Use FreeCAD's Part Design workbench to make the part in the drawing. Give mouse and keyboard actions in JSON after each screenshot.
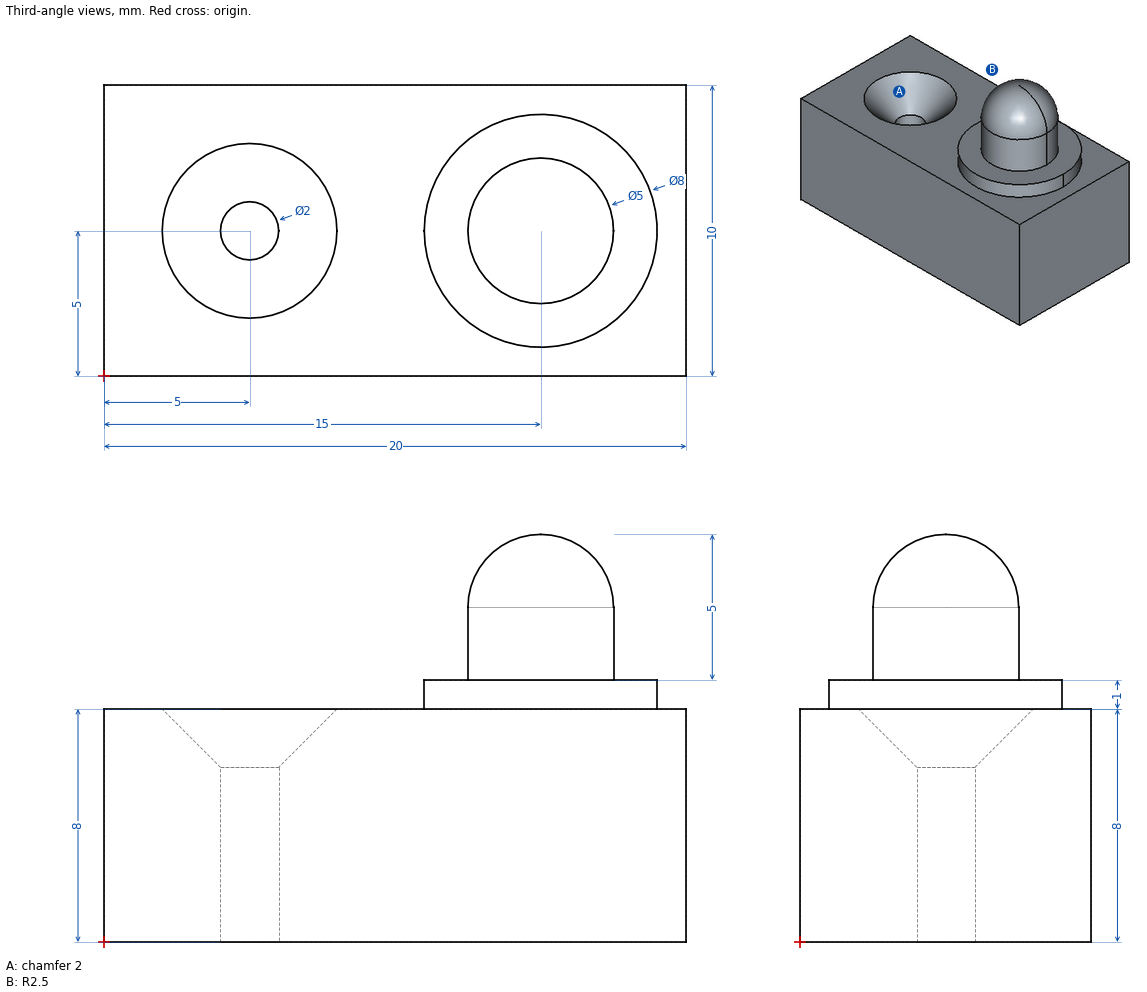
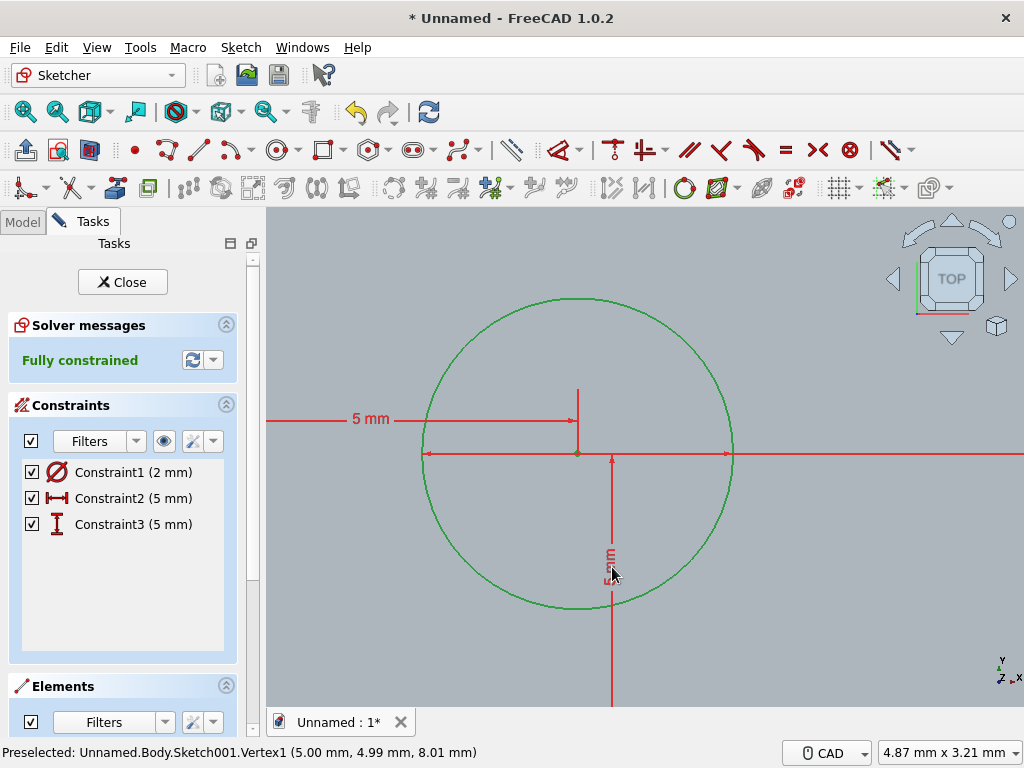
{"action": "left_click", "coordinate": [123, 282]}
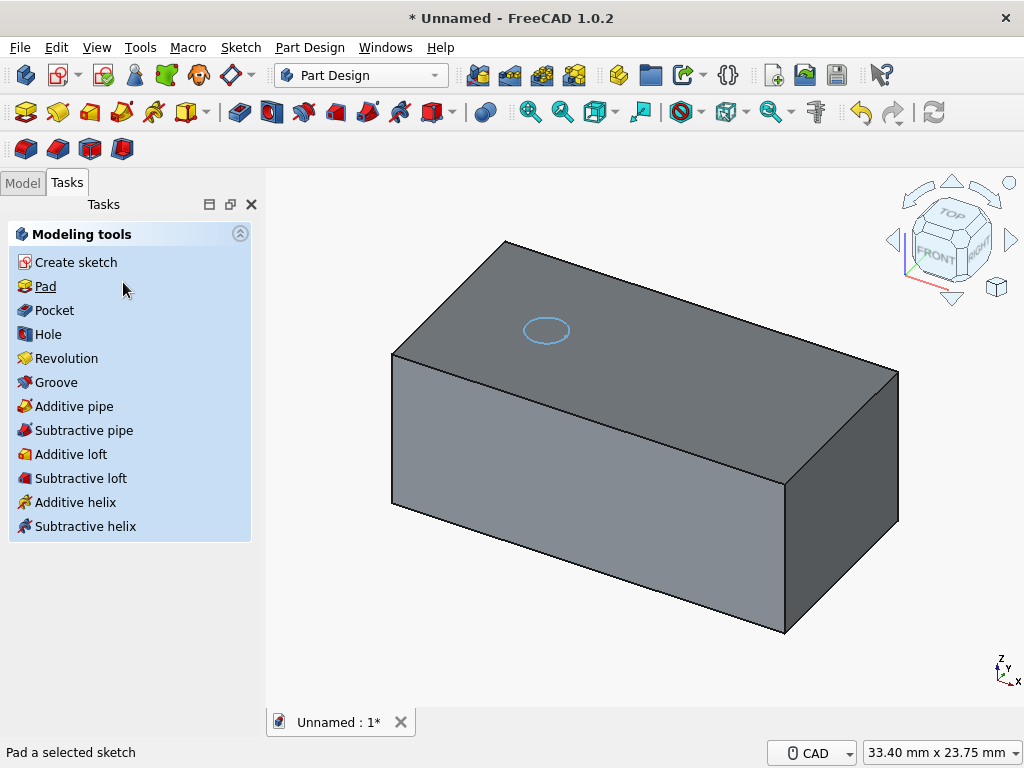
{"action": "left_click", "coordinate": [240, 112]}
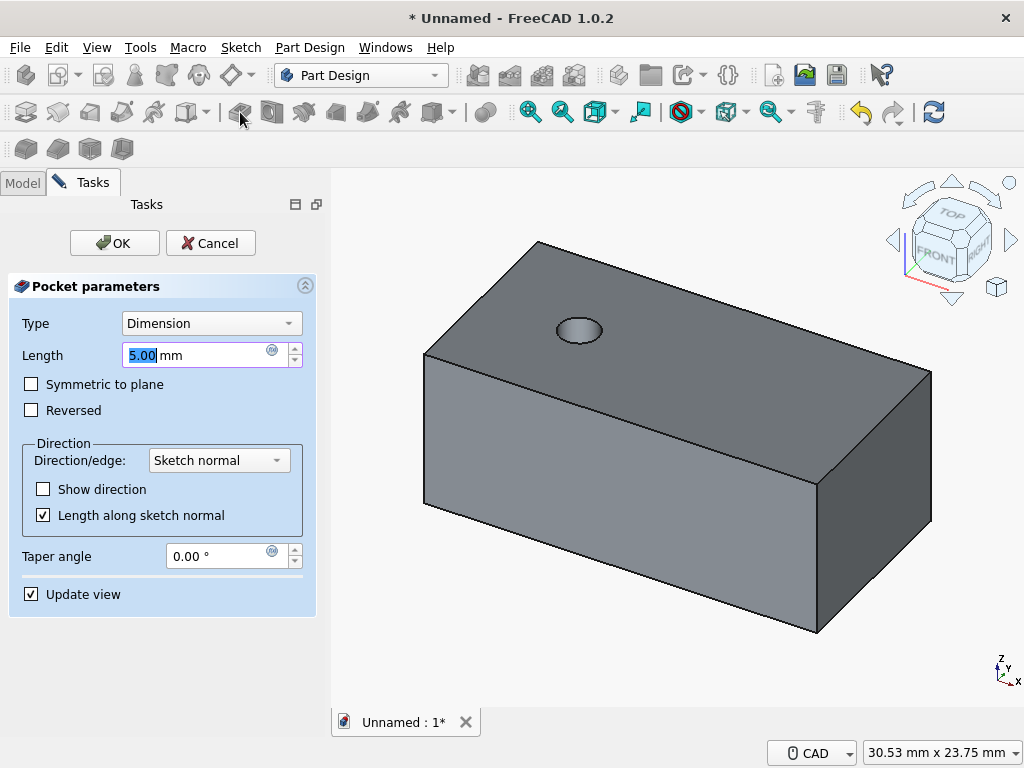
{"action": "type", "text": "8"}
{"action": "key", "text": "Tab"}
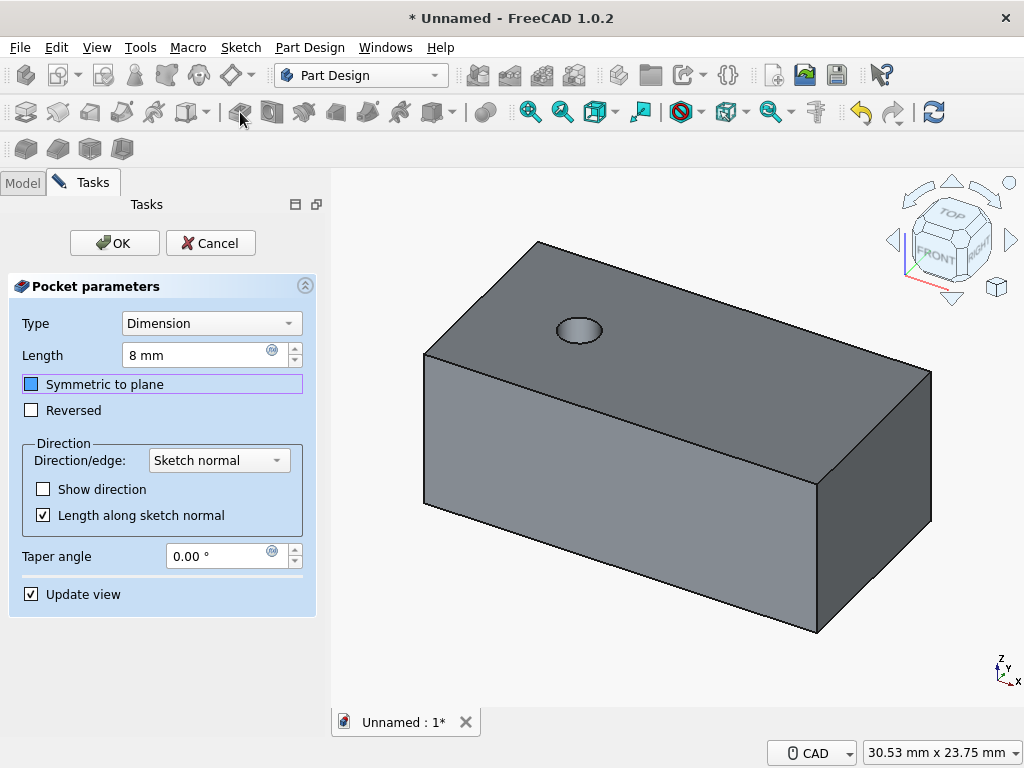
{"action": "left_click", "coordinate": [115, 243]}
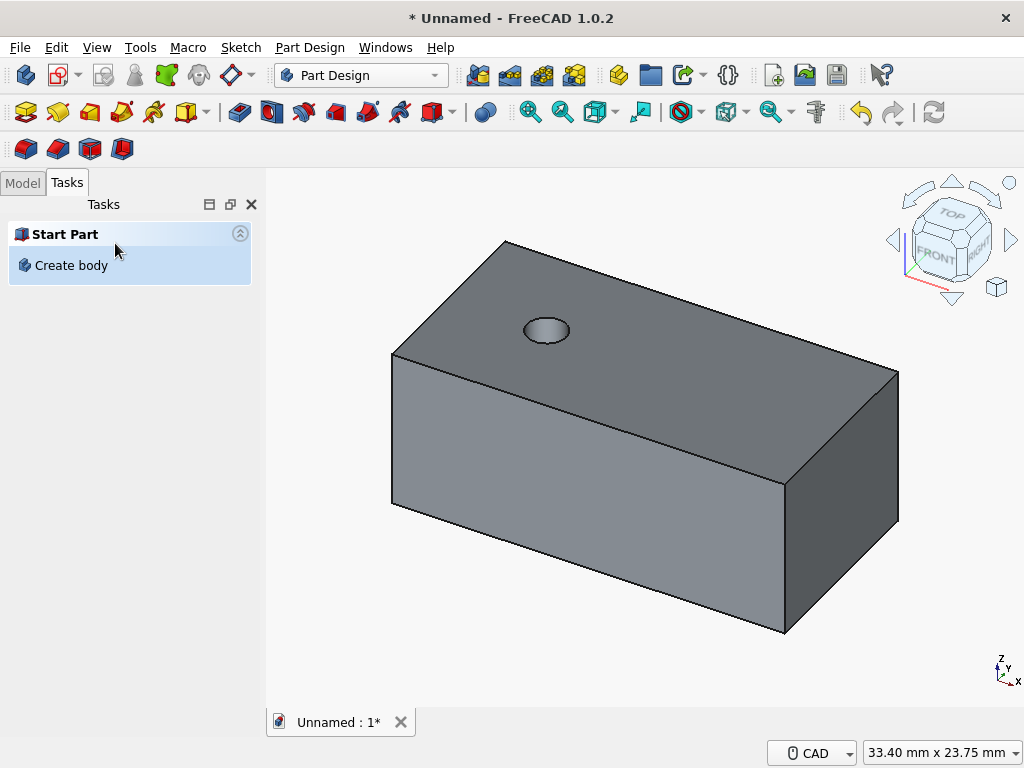
{"action": "left_click", "coordinate": [527, 323]}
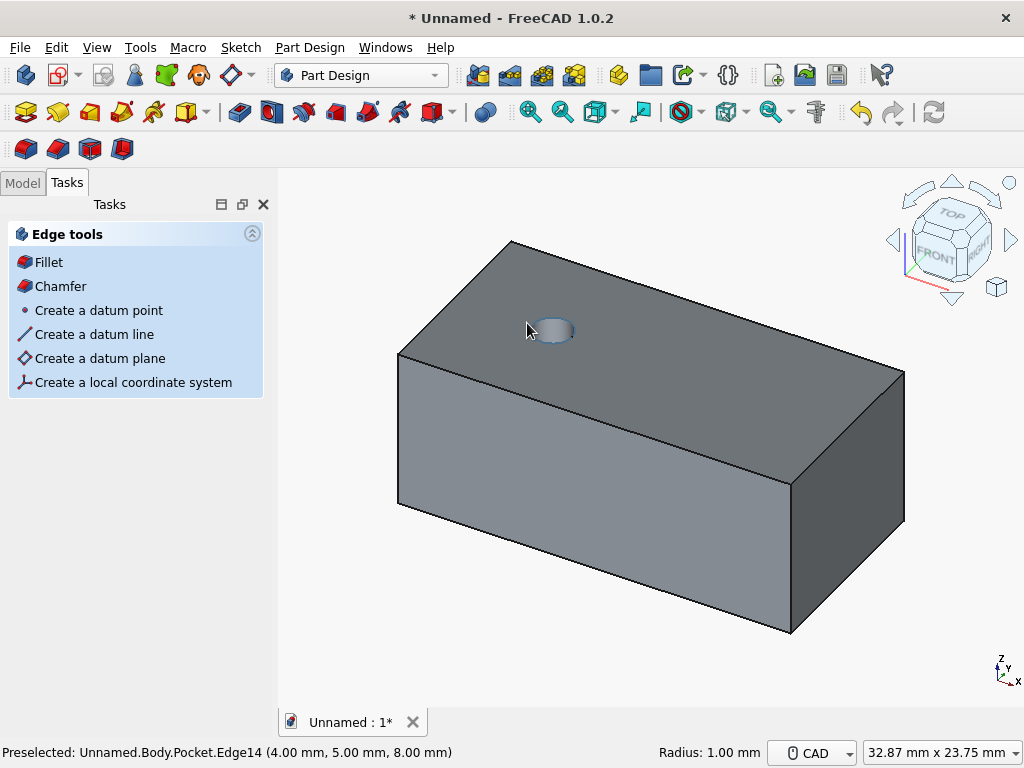
{"action": "left_click", "coordinate": [58, 150]}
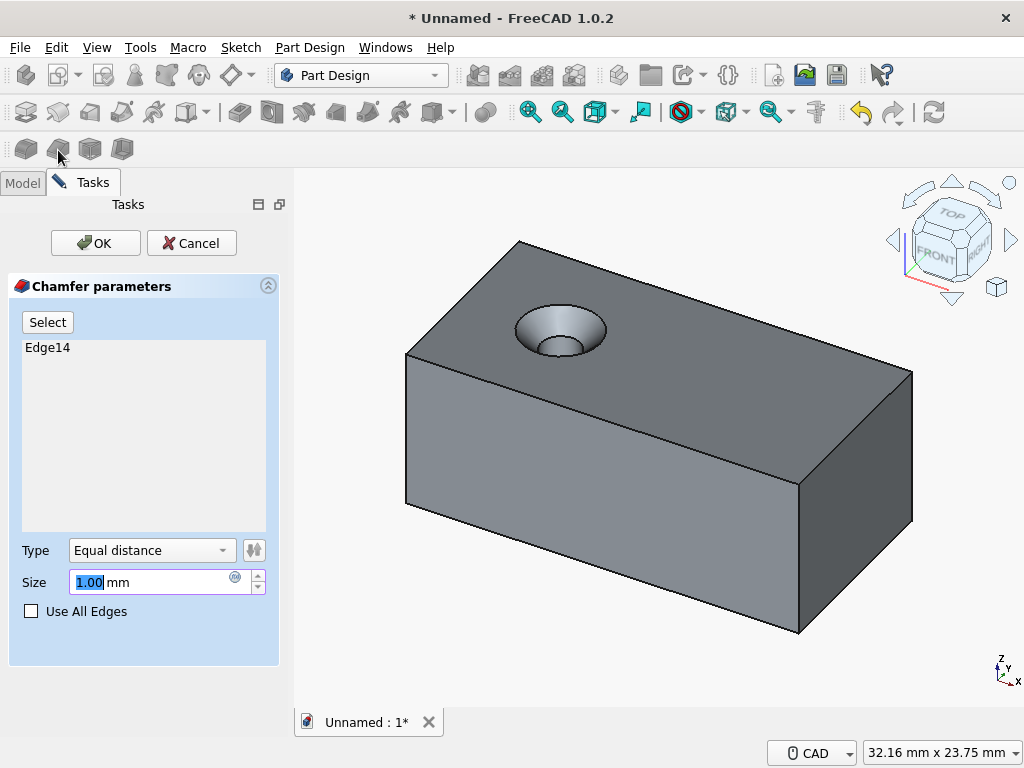
{"action": "type", "text": "2"}
{"action": "key", "text": "Tab"}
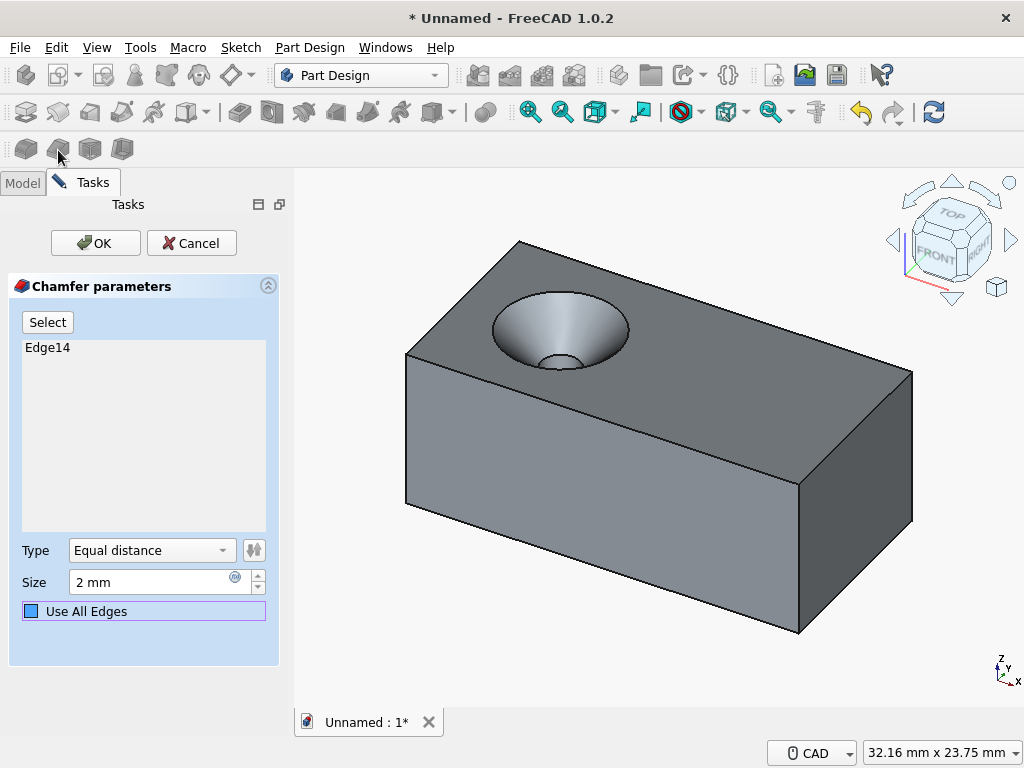
{"action": "left_click", "coordinate": [96, 243]}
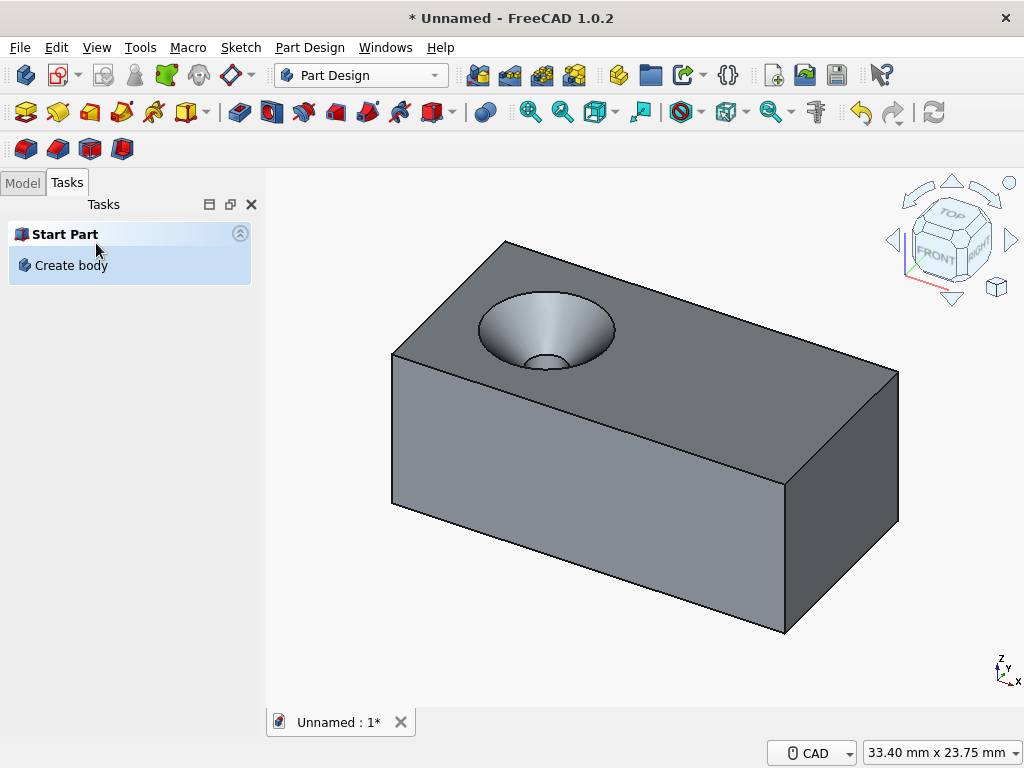
{"action": "left_click", "coordinate": [701, 381]}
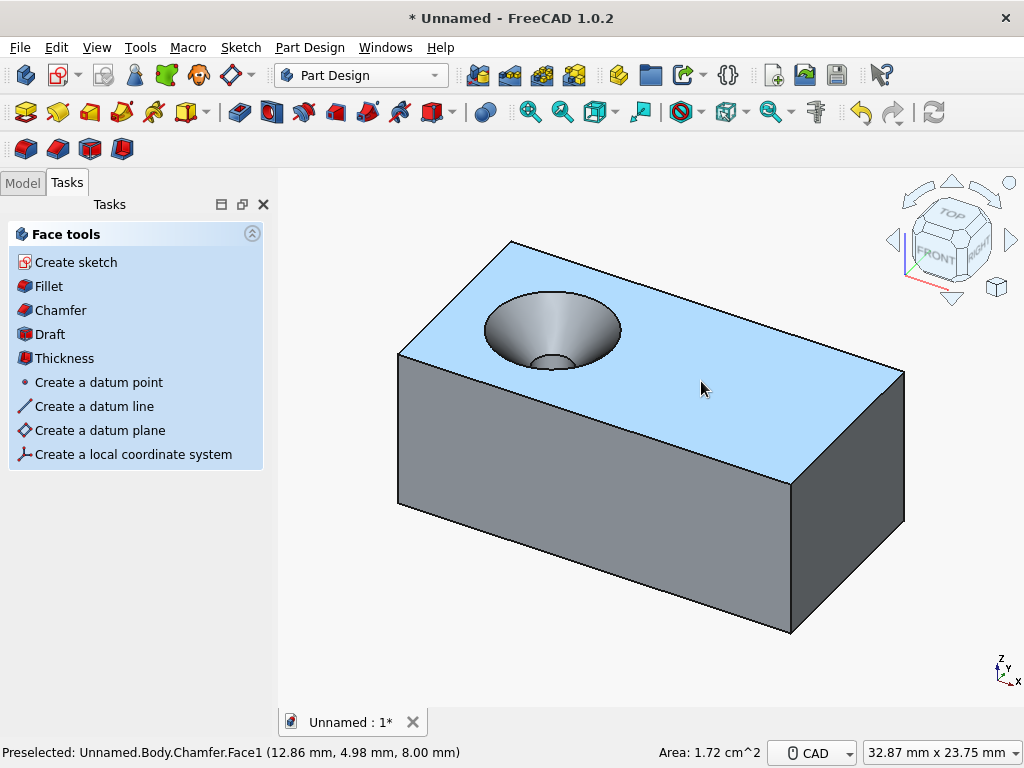
{"action": "left_click", "coordinate": [58, 76]}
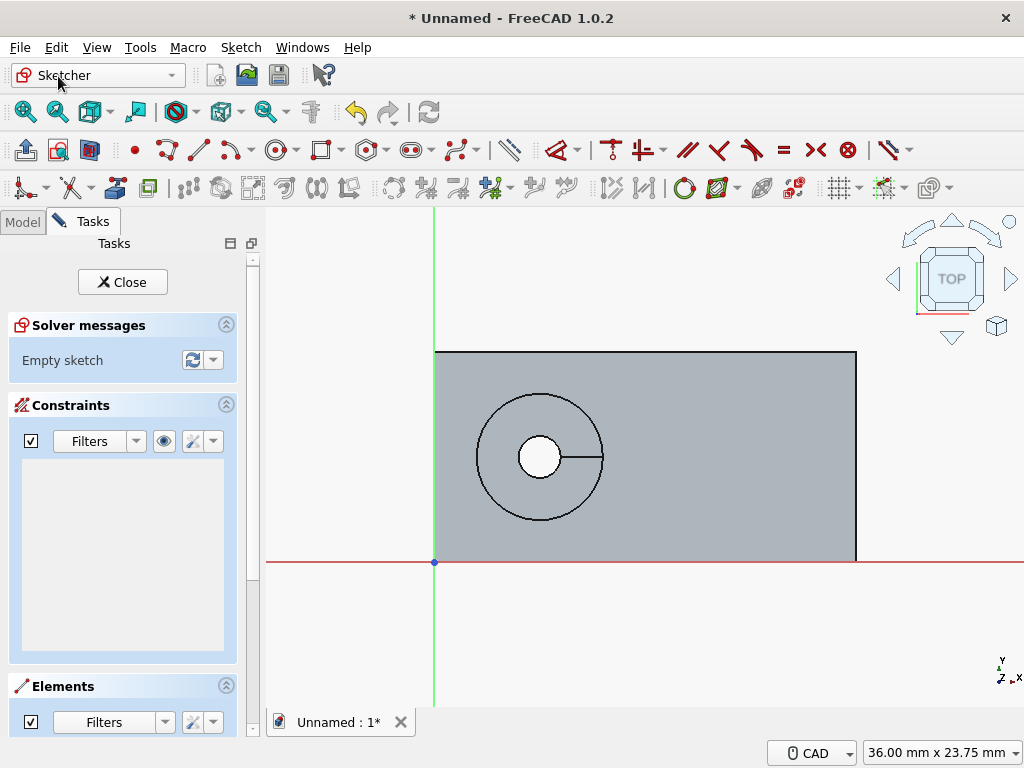
{"action": "scroll", "coordinate": [315, 409], "scroll_direction": "down", "scroll_amount": 1}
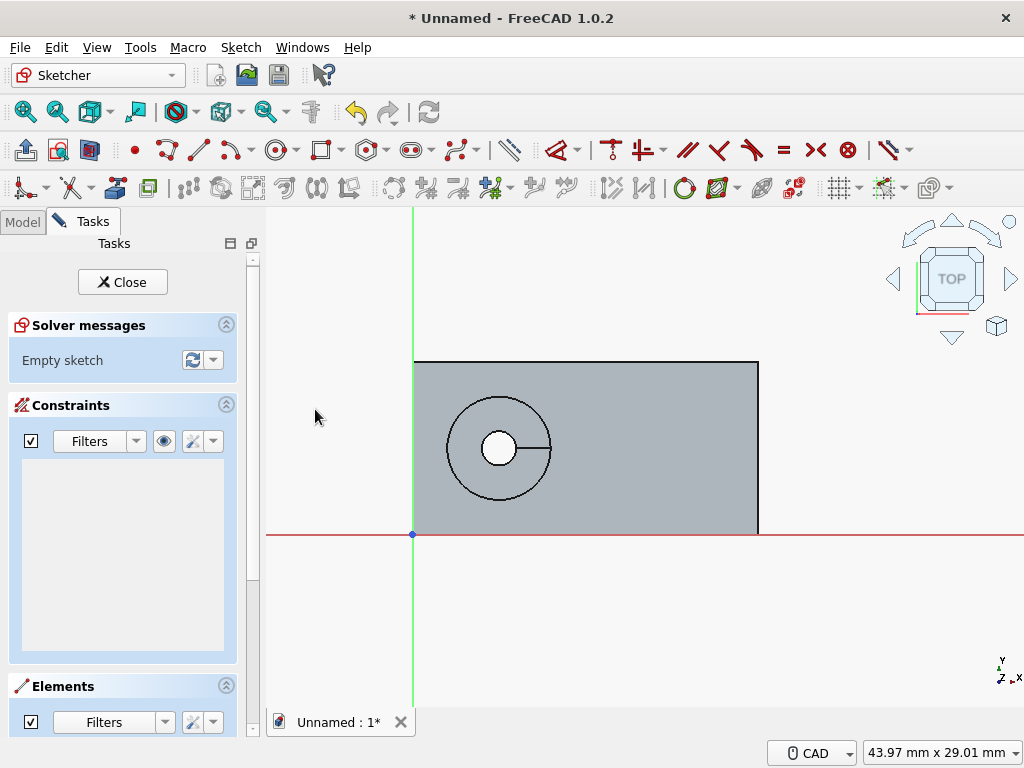
{"action": "left_click", "coordinate": [276, 150]}